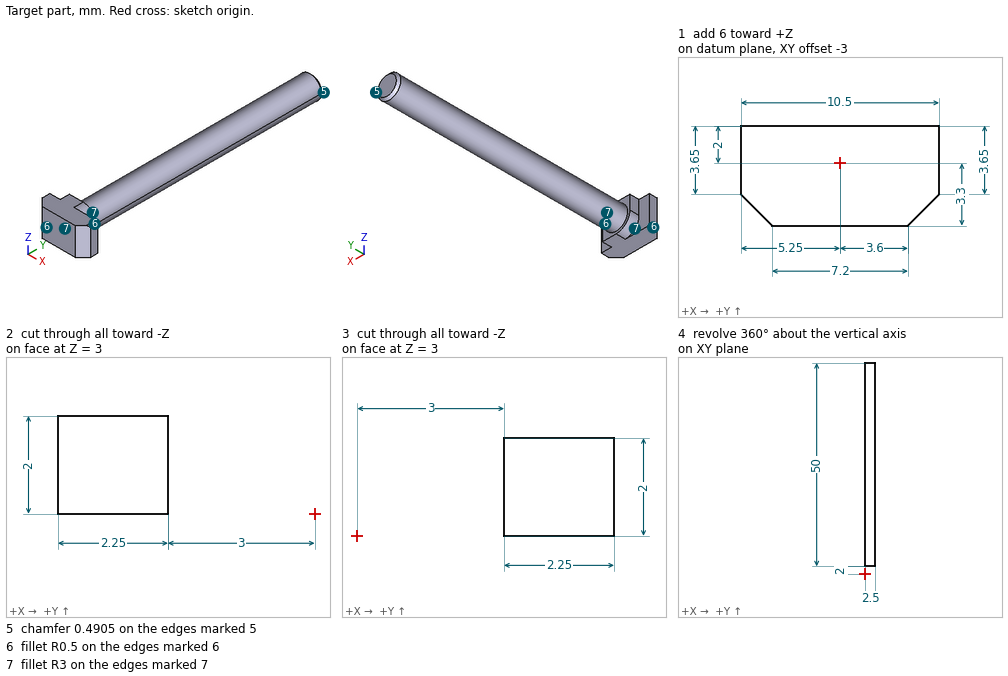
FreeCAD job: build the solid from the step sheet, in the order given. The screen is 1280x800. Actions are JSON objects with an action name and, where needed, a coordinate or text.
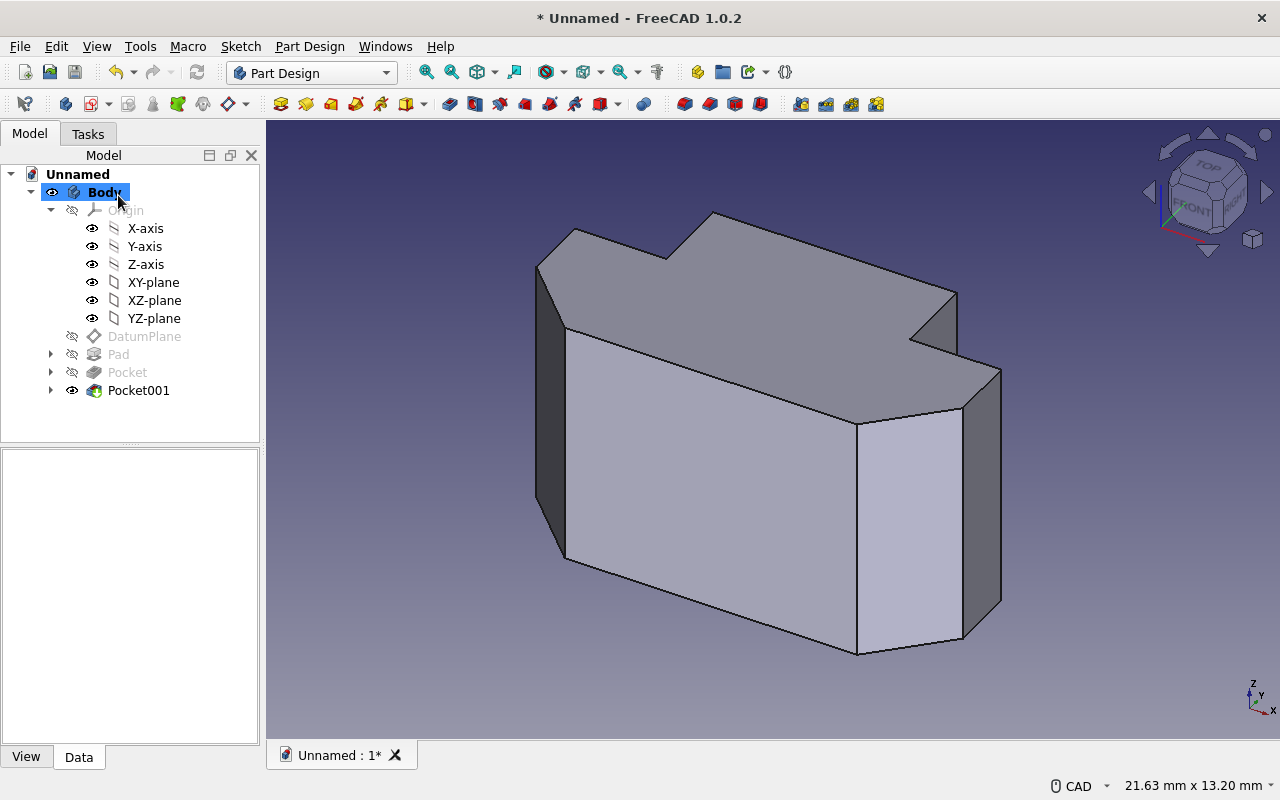
{"action": "left_click", "coordinate": [90, 104]}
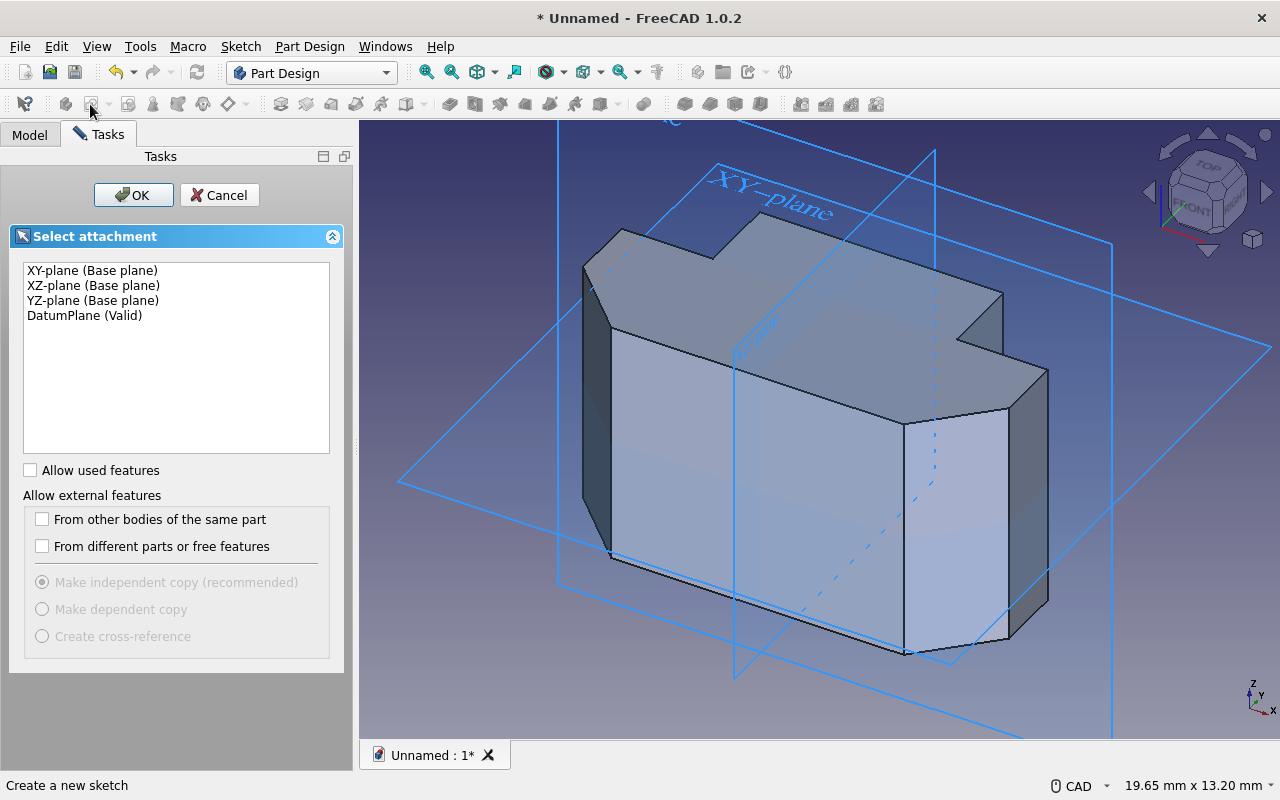
{"action": "left_click", "coordinate": [84, 270]}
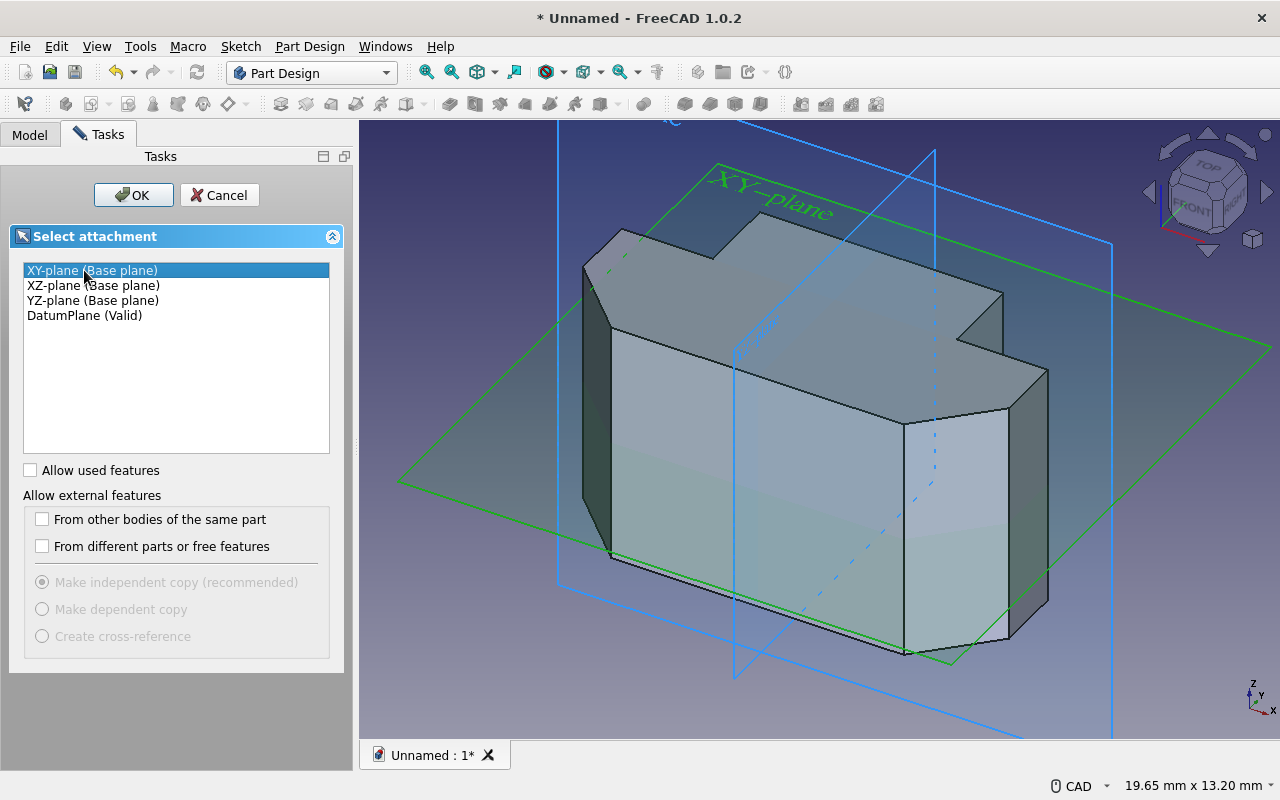
{"action": "left_click", "coordinate": [134, 195]}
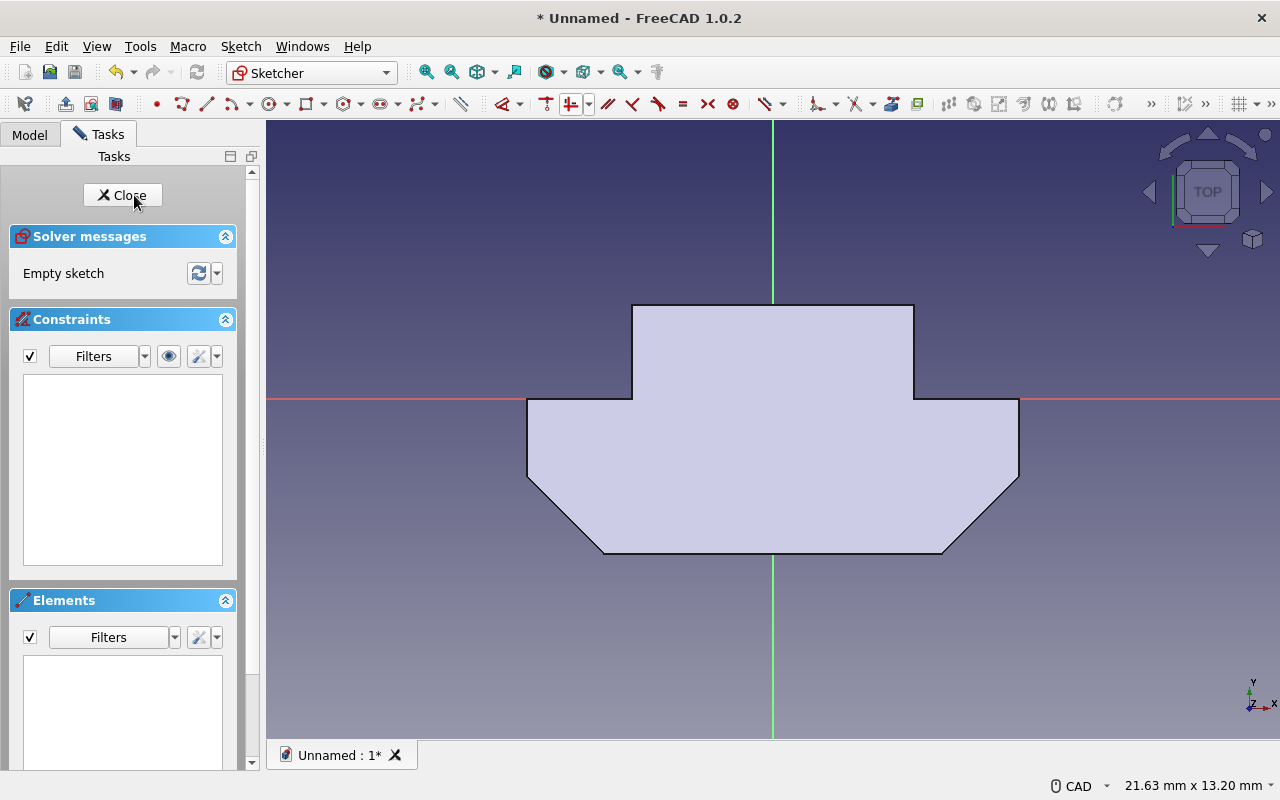
{"action": "key", "text": "q s"}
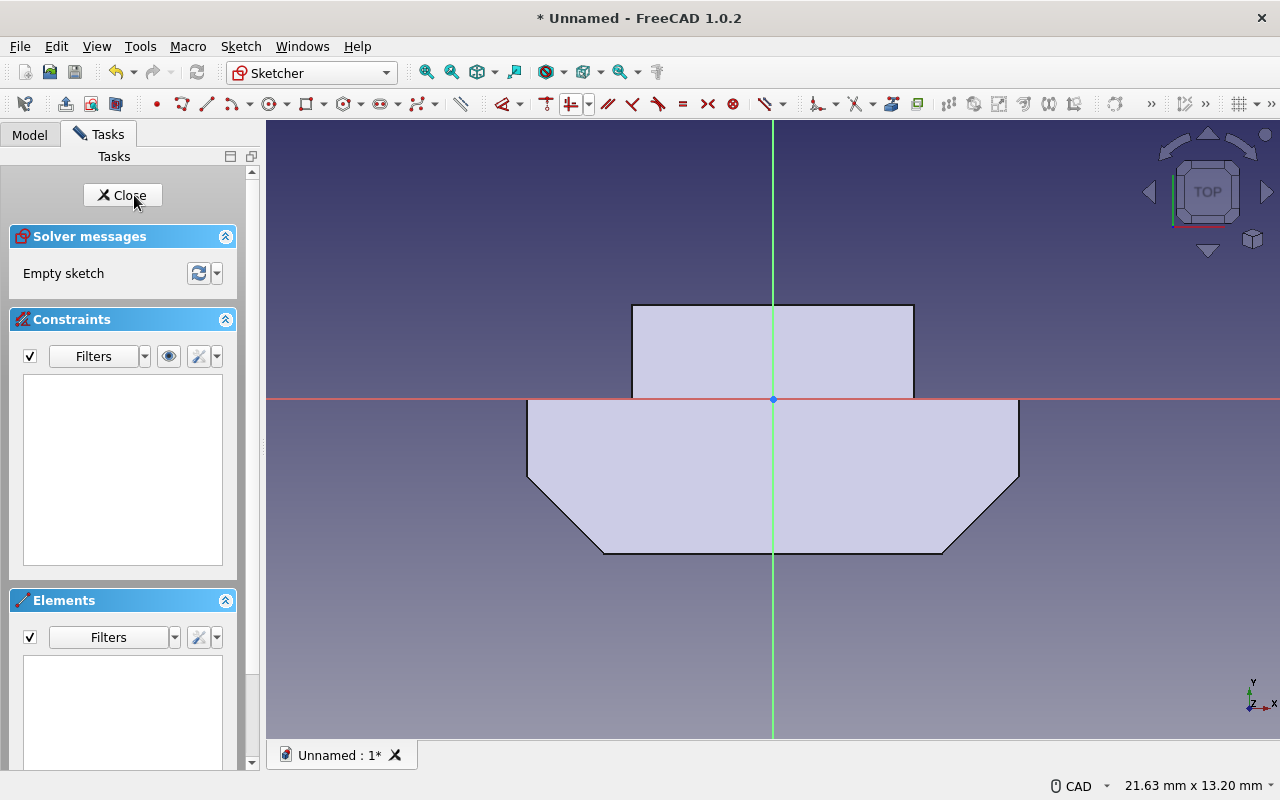
{"action": "scroll", "coordinate": [679, 677], "scroll_direction": "down", "scroll_amount": 9}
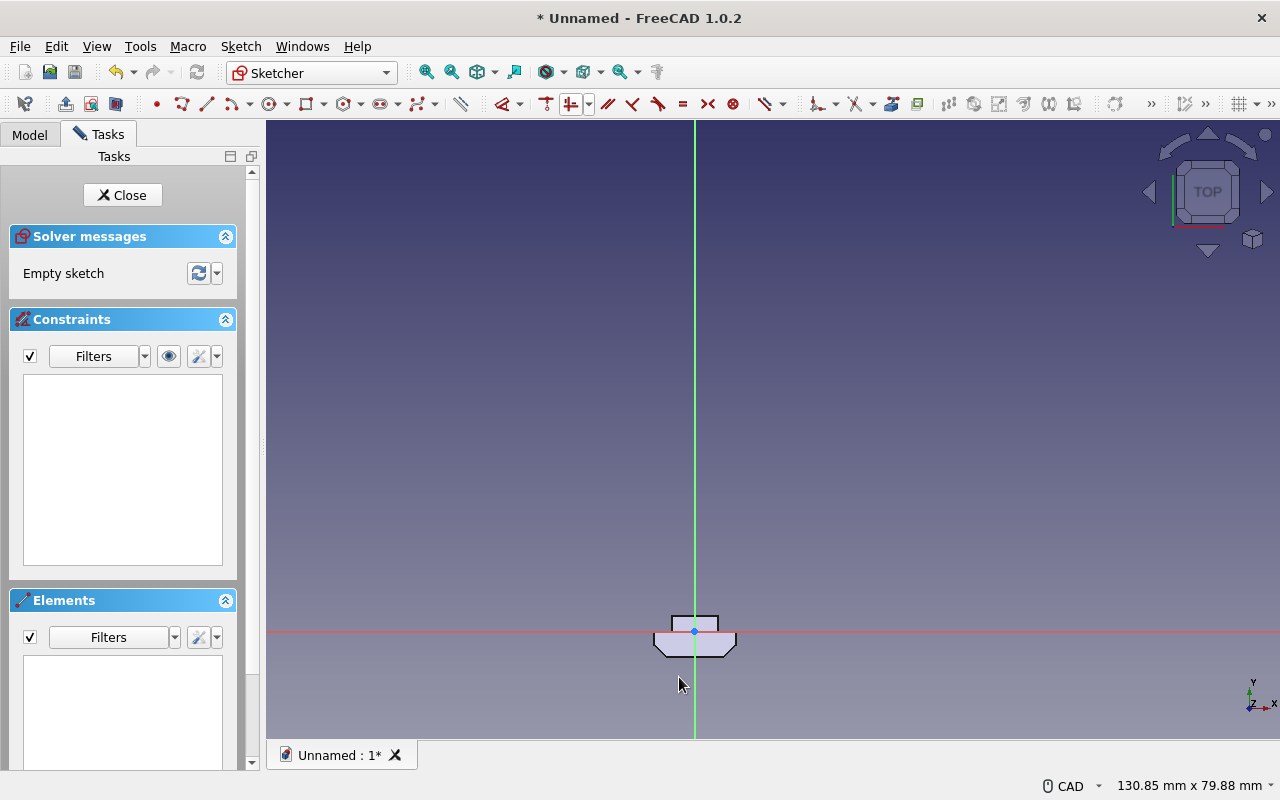
{"action": "left_click", "coordinate": [306, 104]}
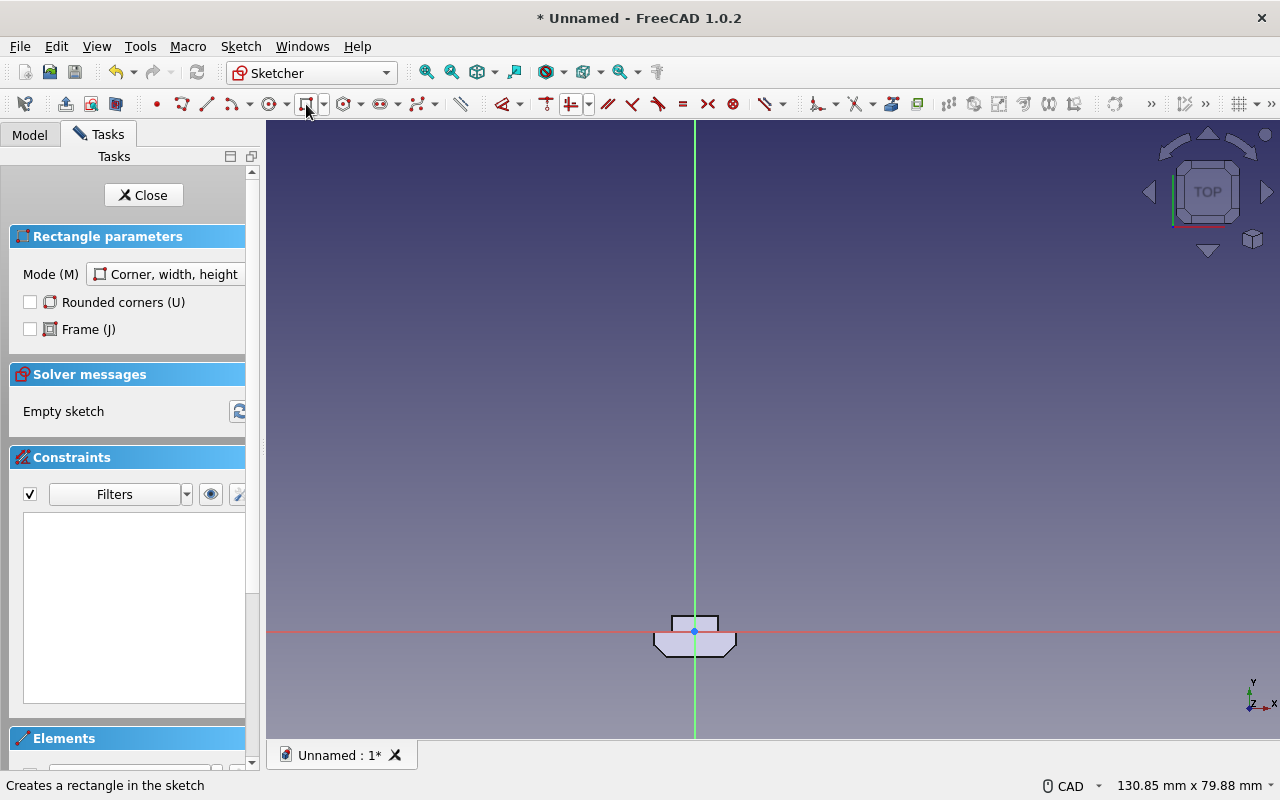
{"action": "left_click", "coordinate": [695, 229]}
{"action": "left_click", "coordinate": [714, 616]}
{"action": "key", "text": "Escape"}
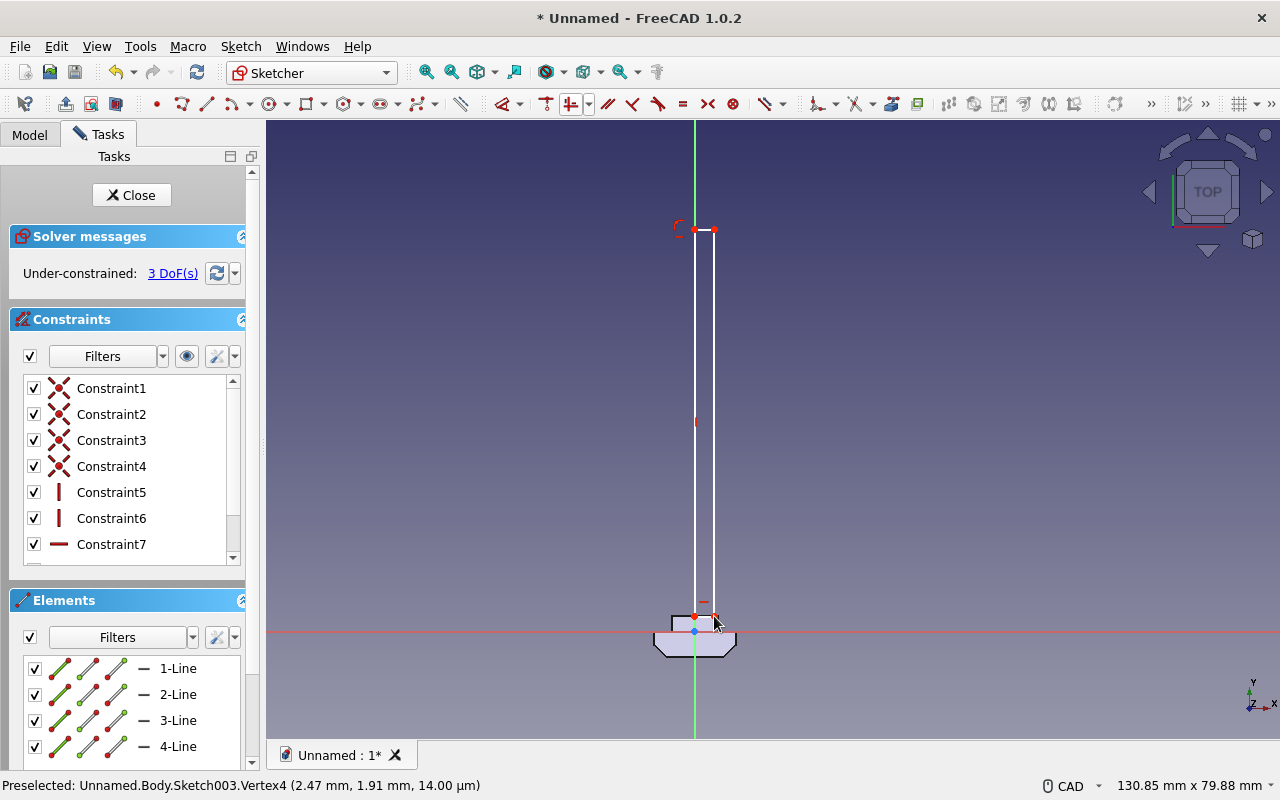
{"action": "left_click", "coordinate": [502, 104]}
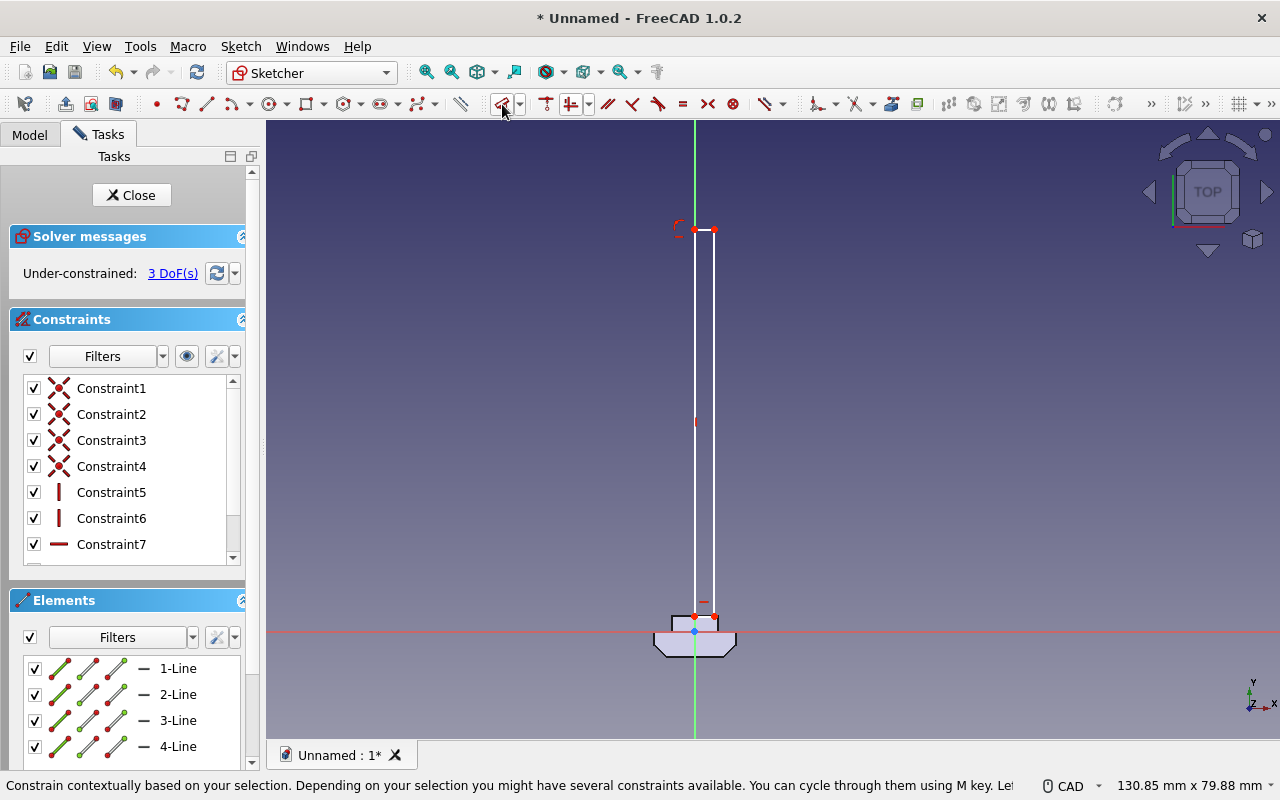
{"action": "left_click", "coordinate": [695, 346]}
{"action": "left_click", "coordinate": [661, 424]}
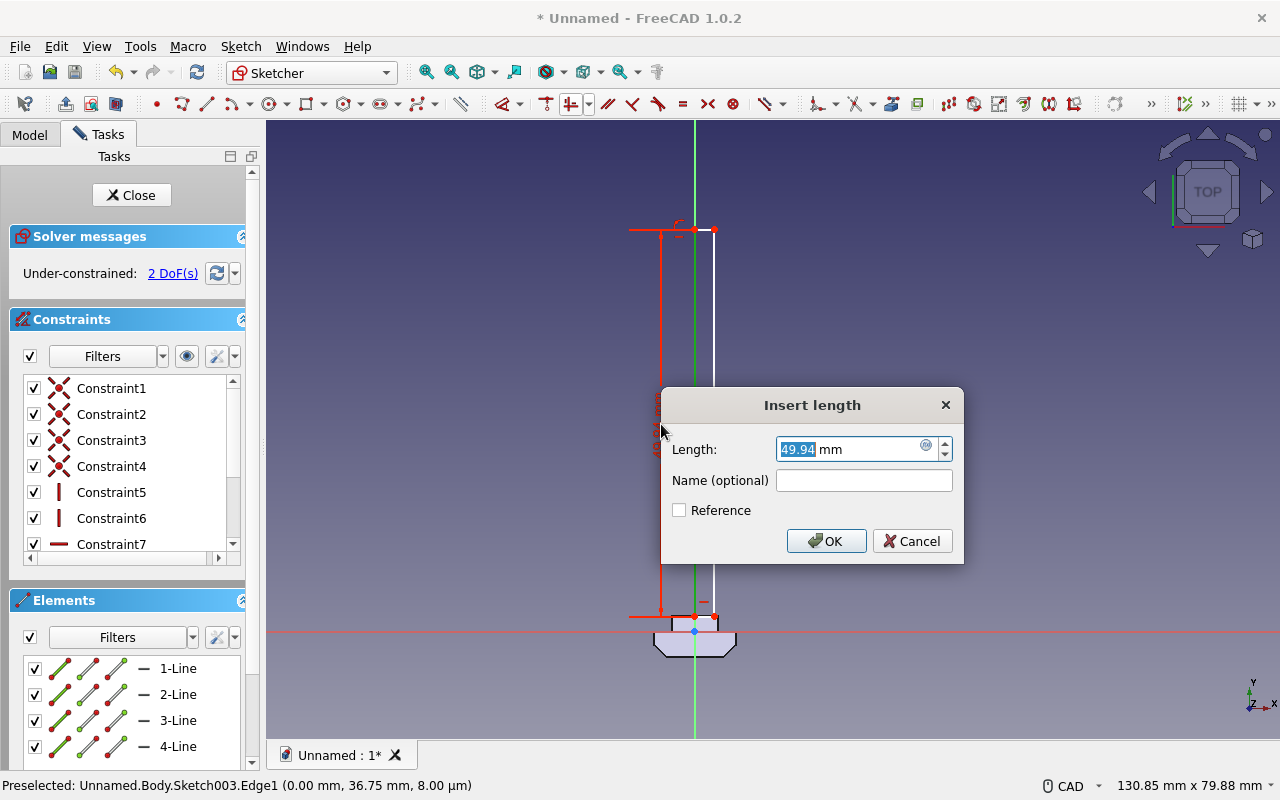
{"action": "type", "text": "50"}
{"action": "key", "text": "Return"}